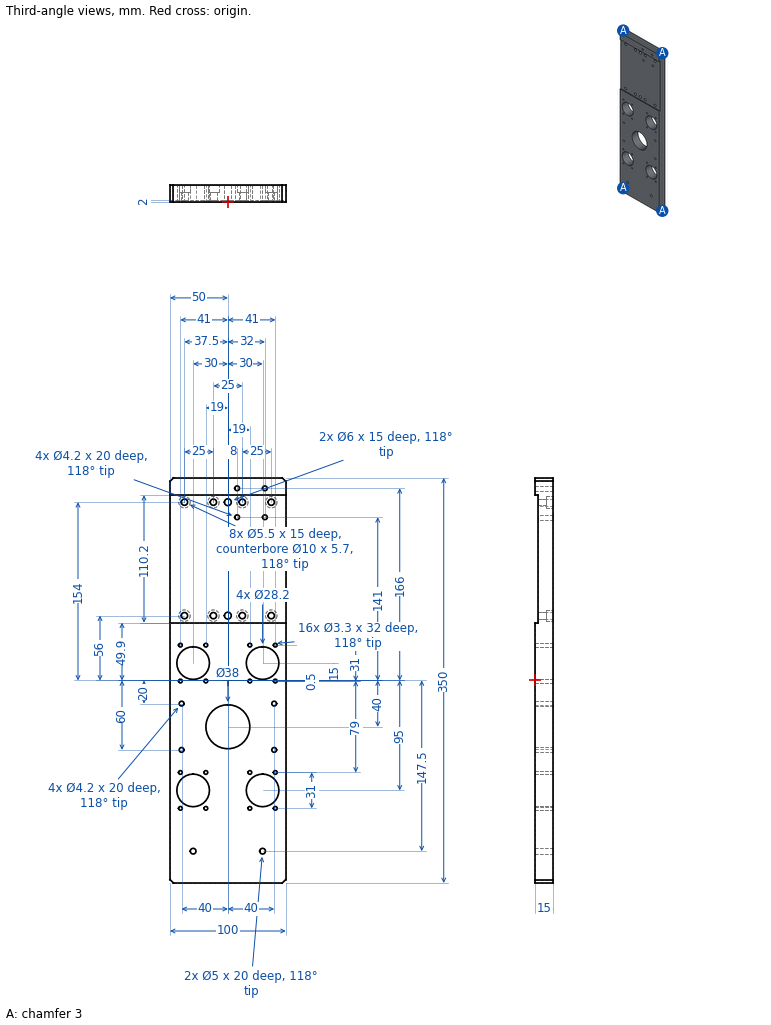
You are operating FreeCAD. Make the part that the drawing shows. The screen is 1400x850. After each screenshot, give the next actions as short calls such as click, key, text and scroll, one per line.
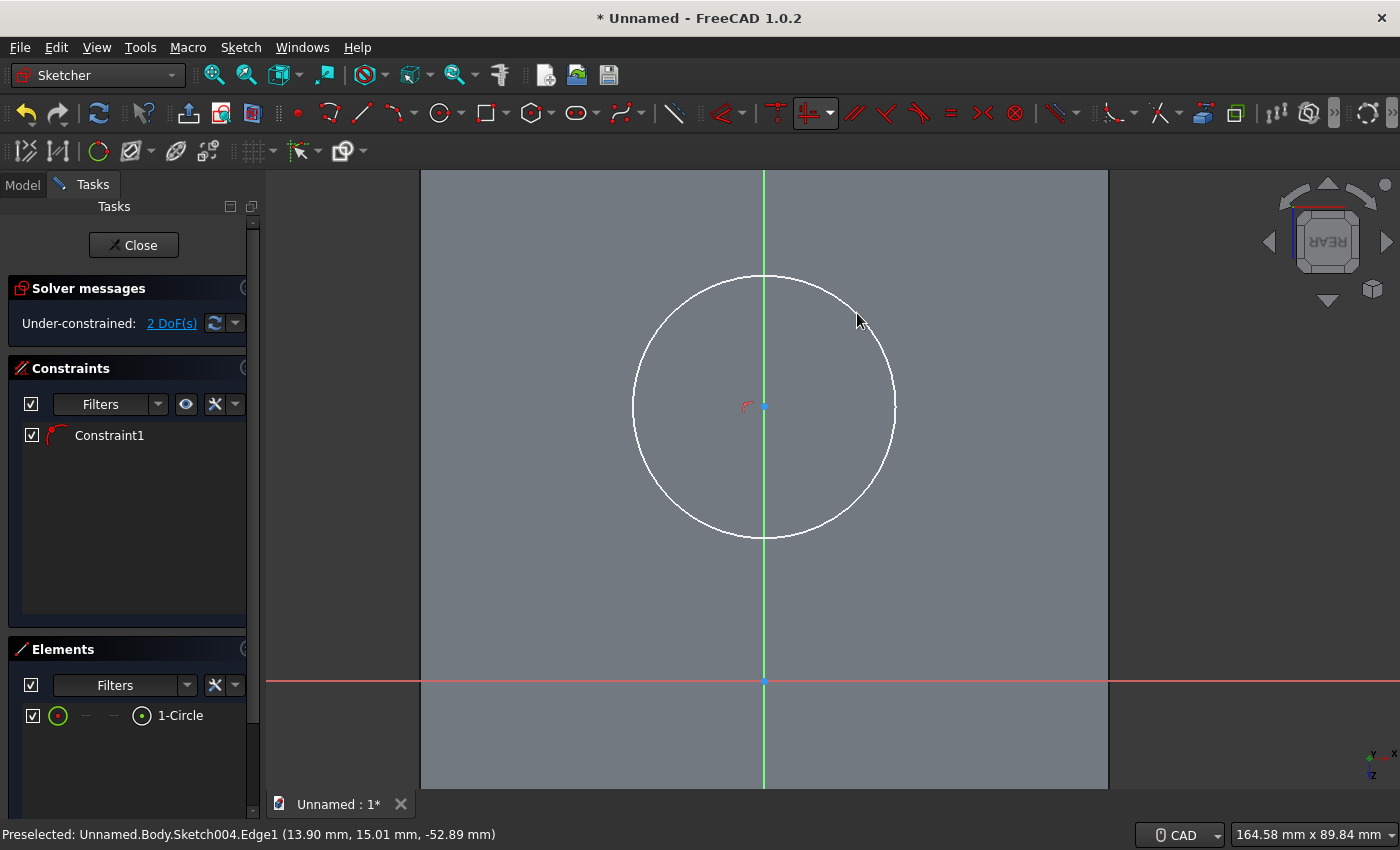
key(d)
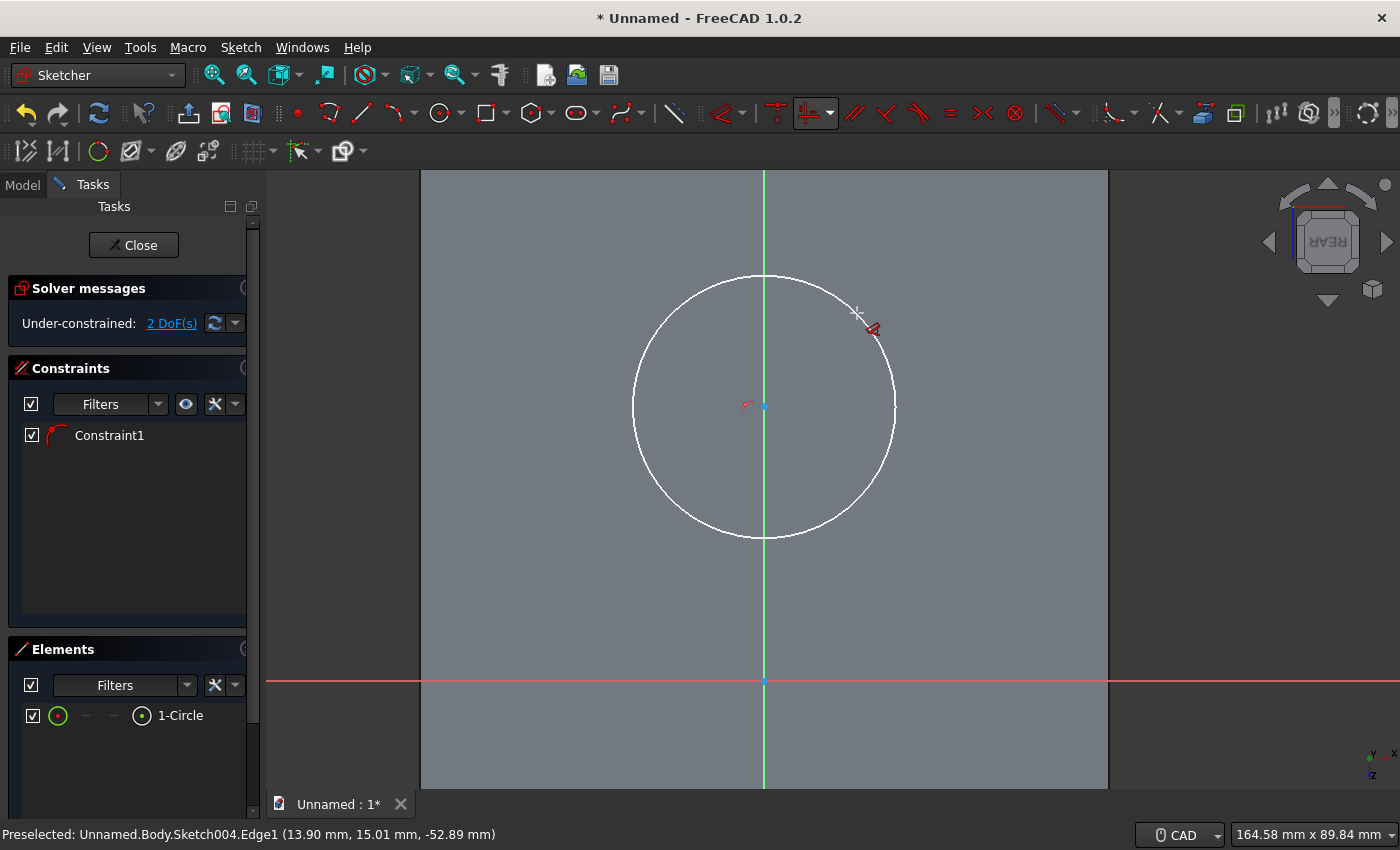
click(857, 314)
click(880, 291)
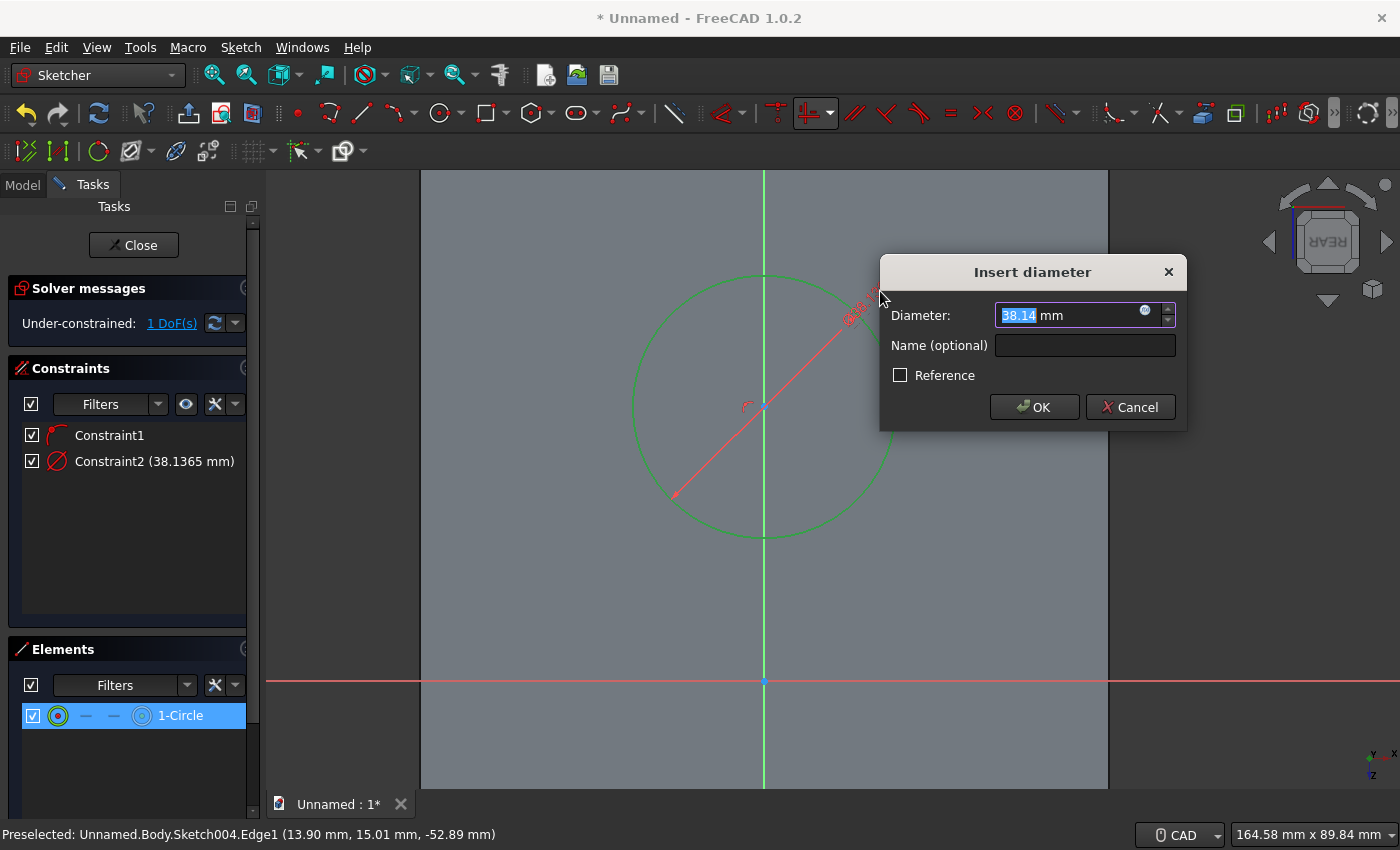
text(38)
key(Return)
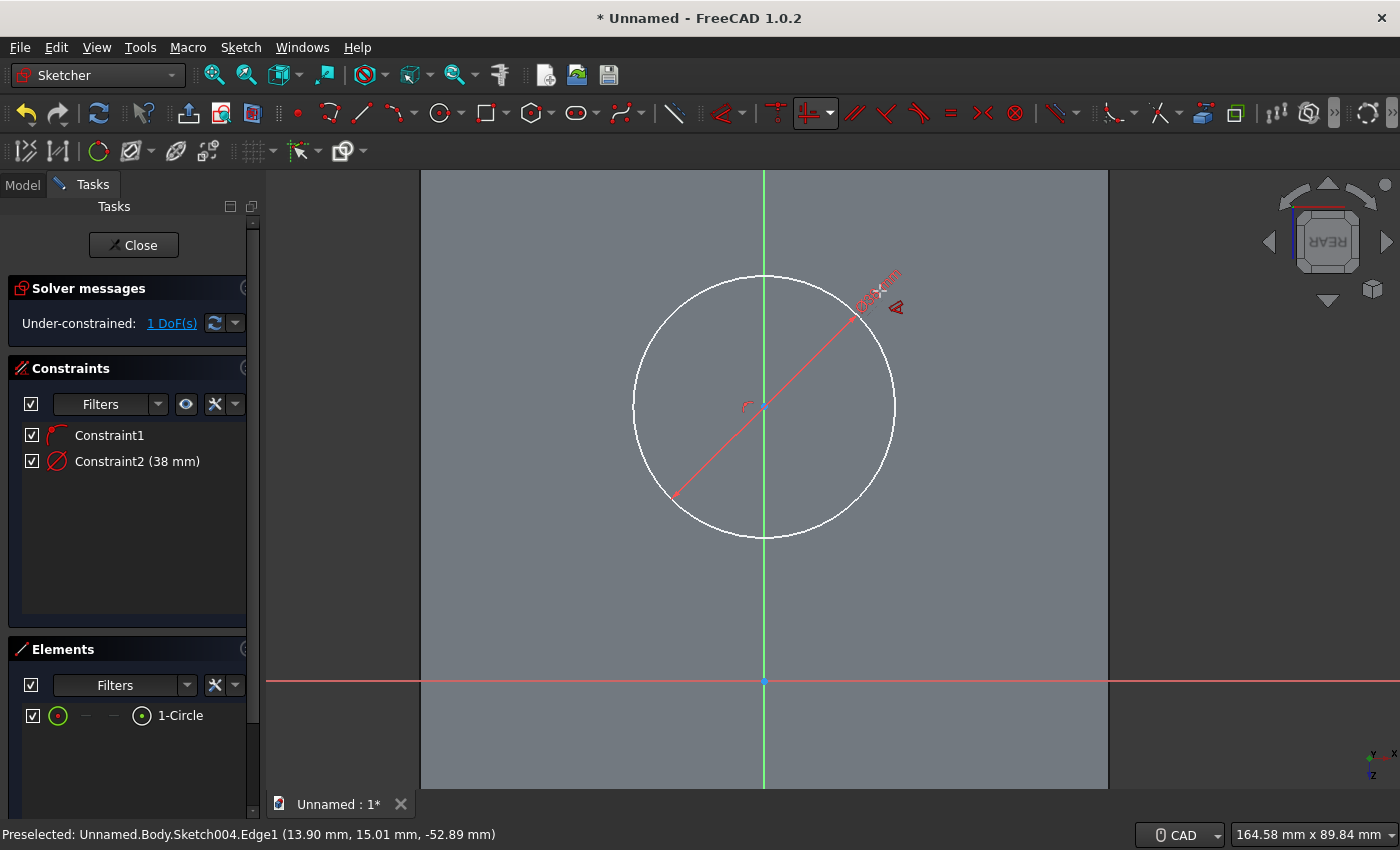
click(764, 407)
click(798, 481)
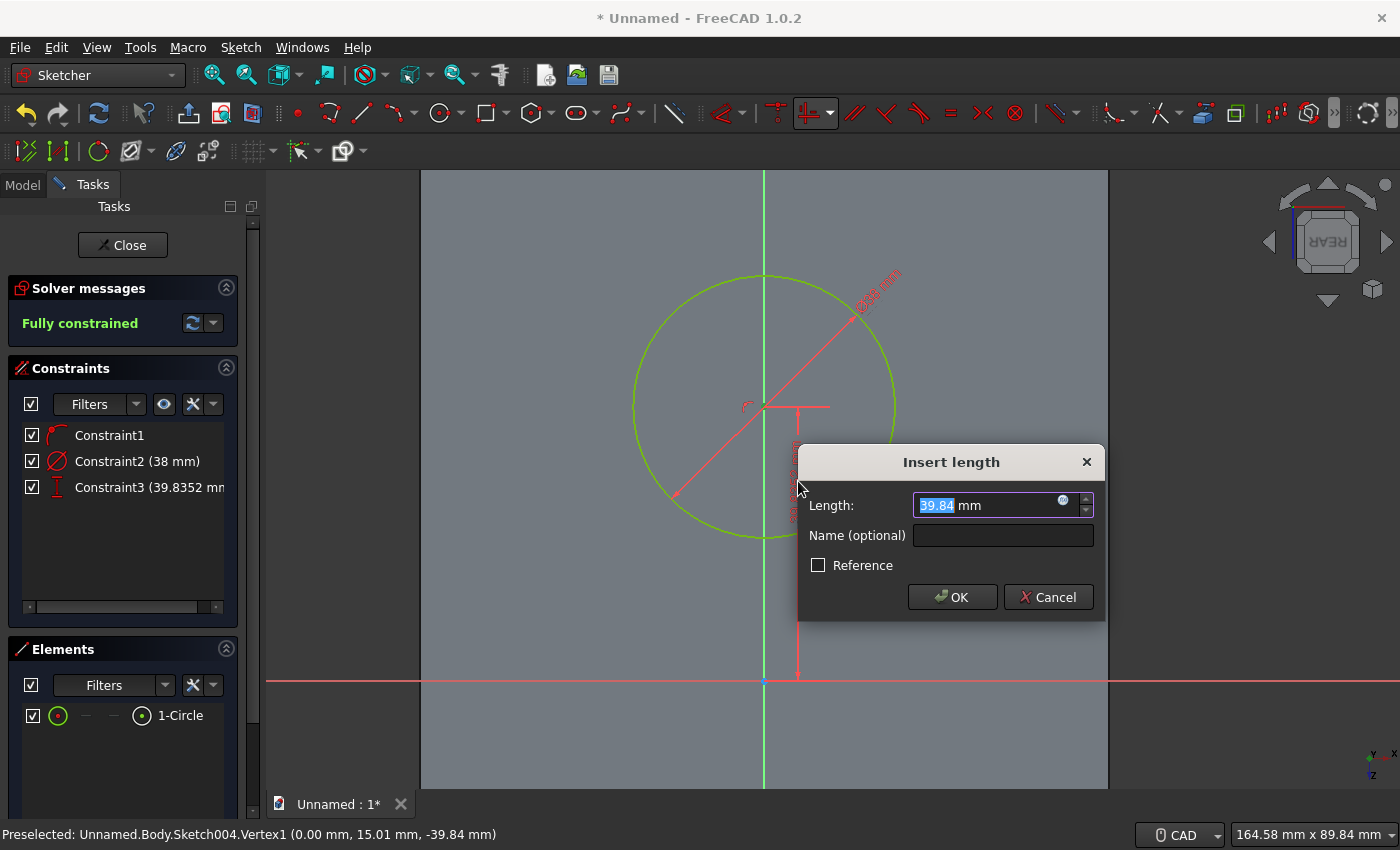
text(40)
key(Return)
key(Escape)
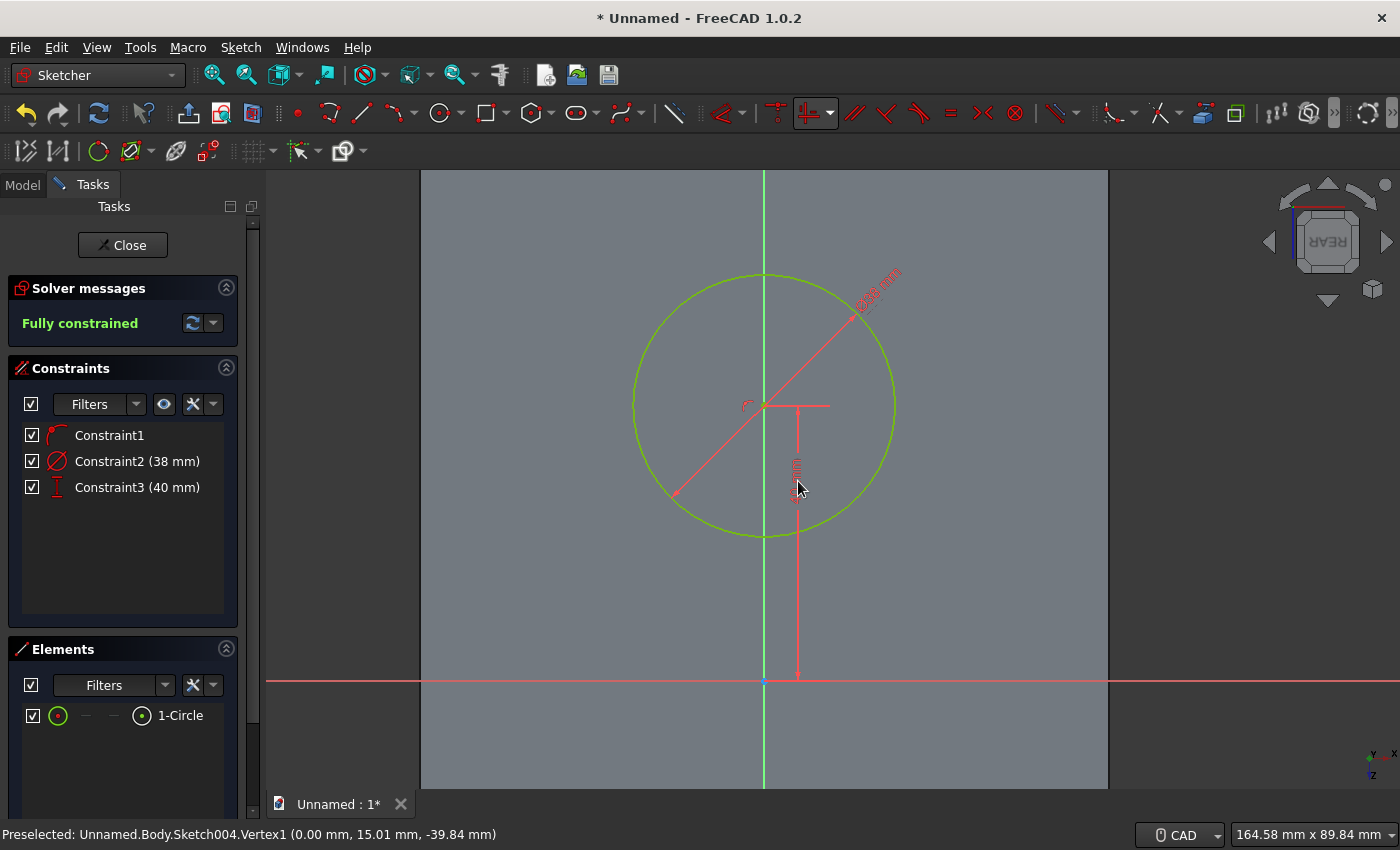
click(123, 245)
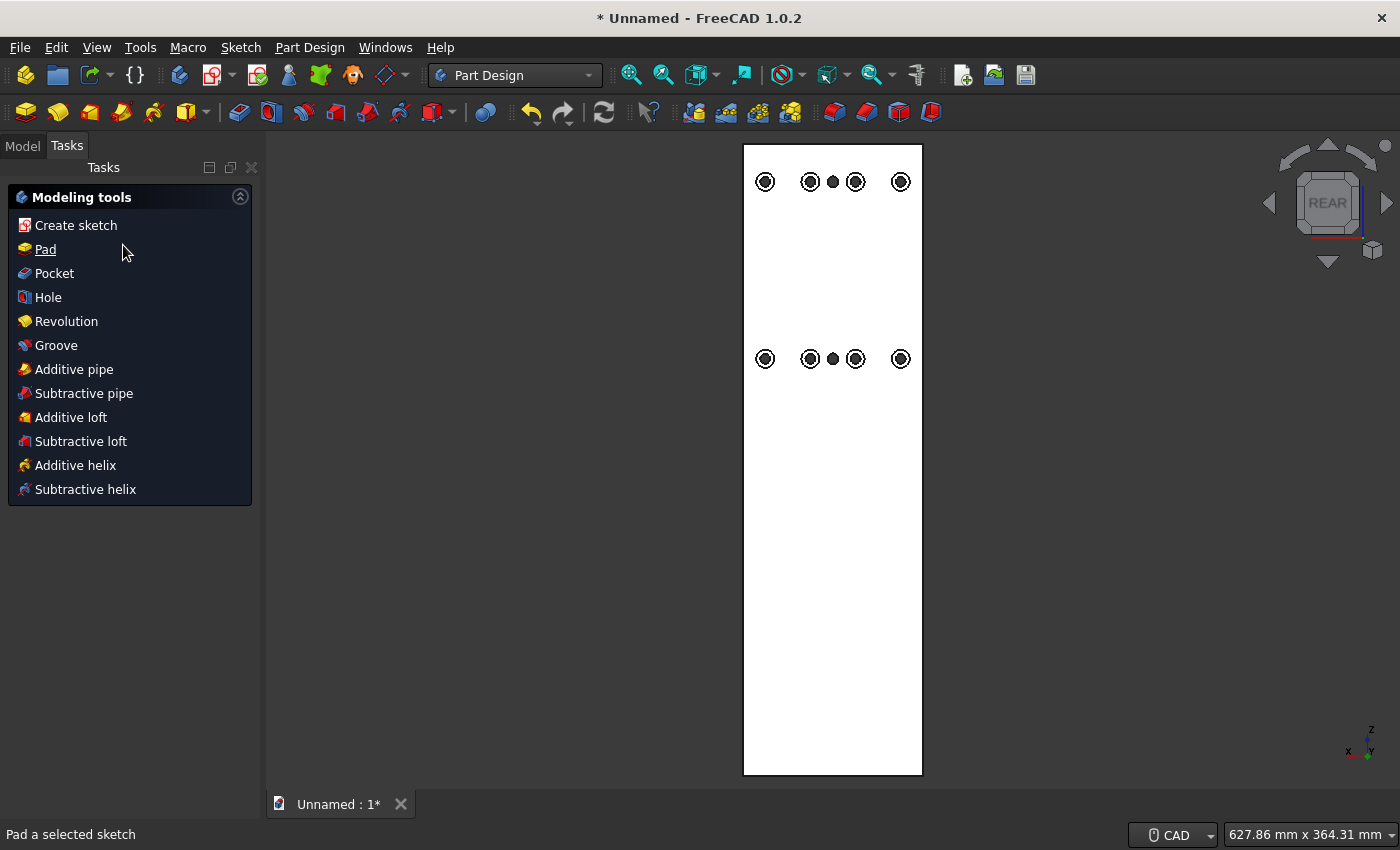
click(240, 112)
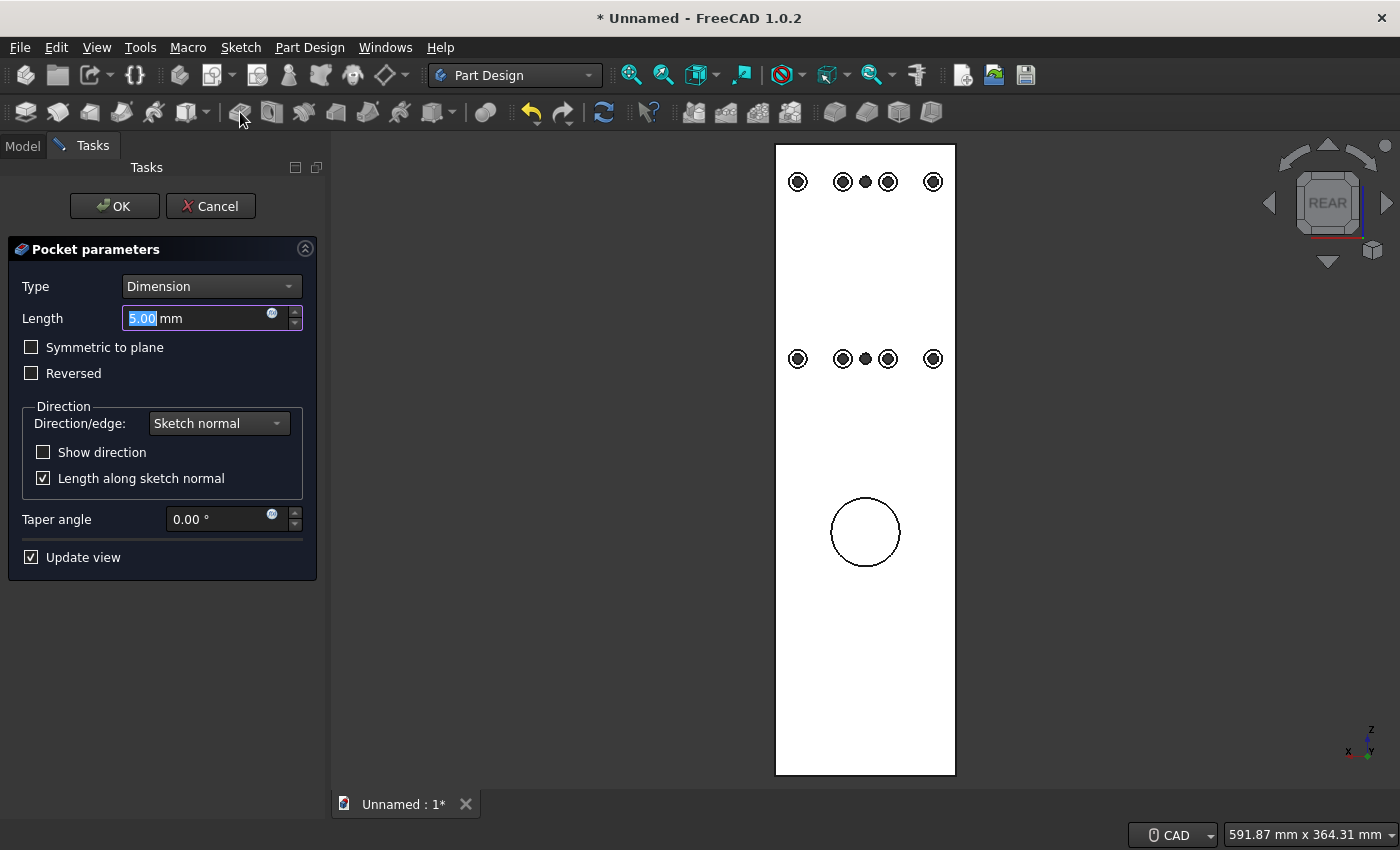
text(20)
key(Tab)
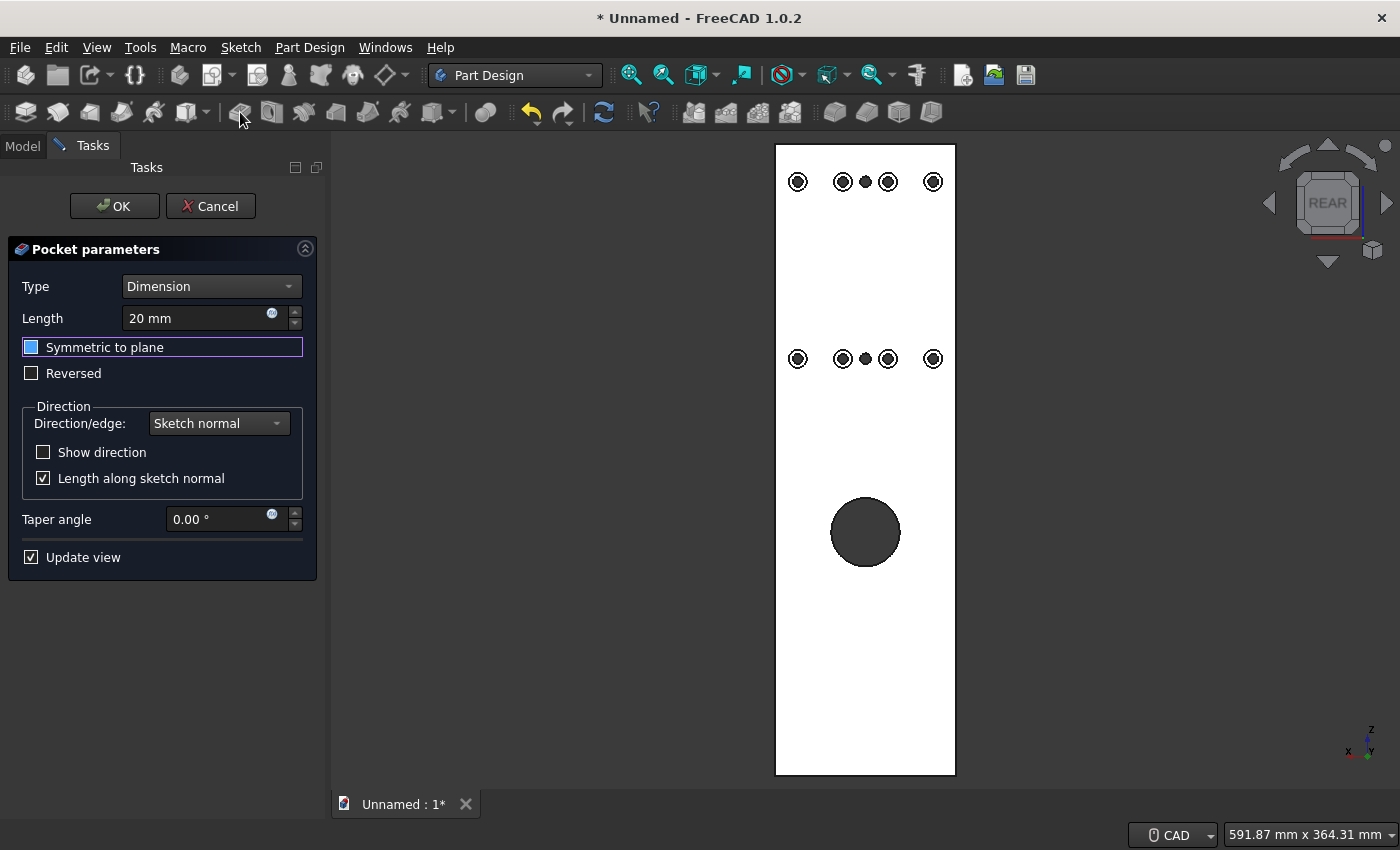
click(115, 206)